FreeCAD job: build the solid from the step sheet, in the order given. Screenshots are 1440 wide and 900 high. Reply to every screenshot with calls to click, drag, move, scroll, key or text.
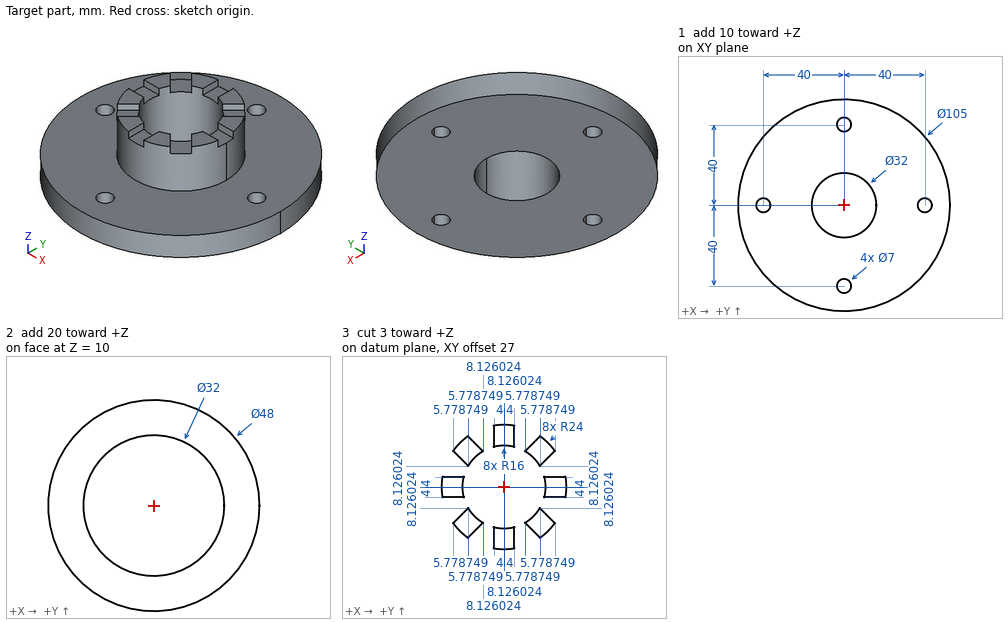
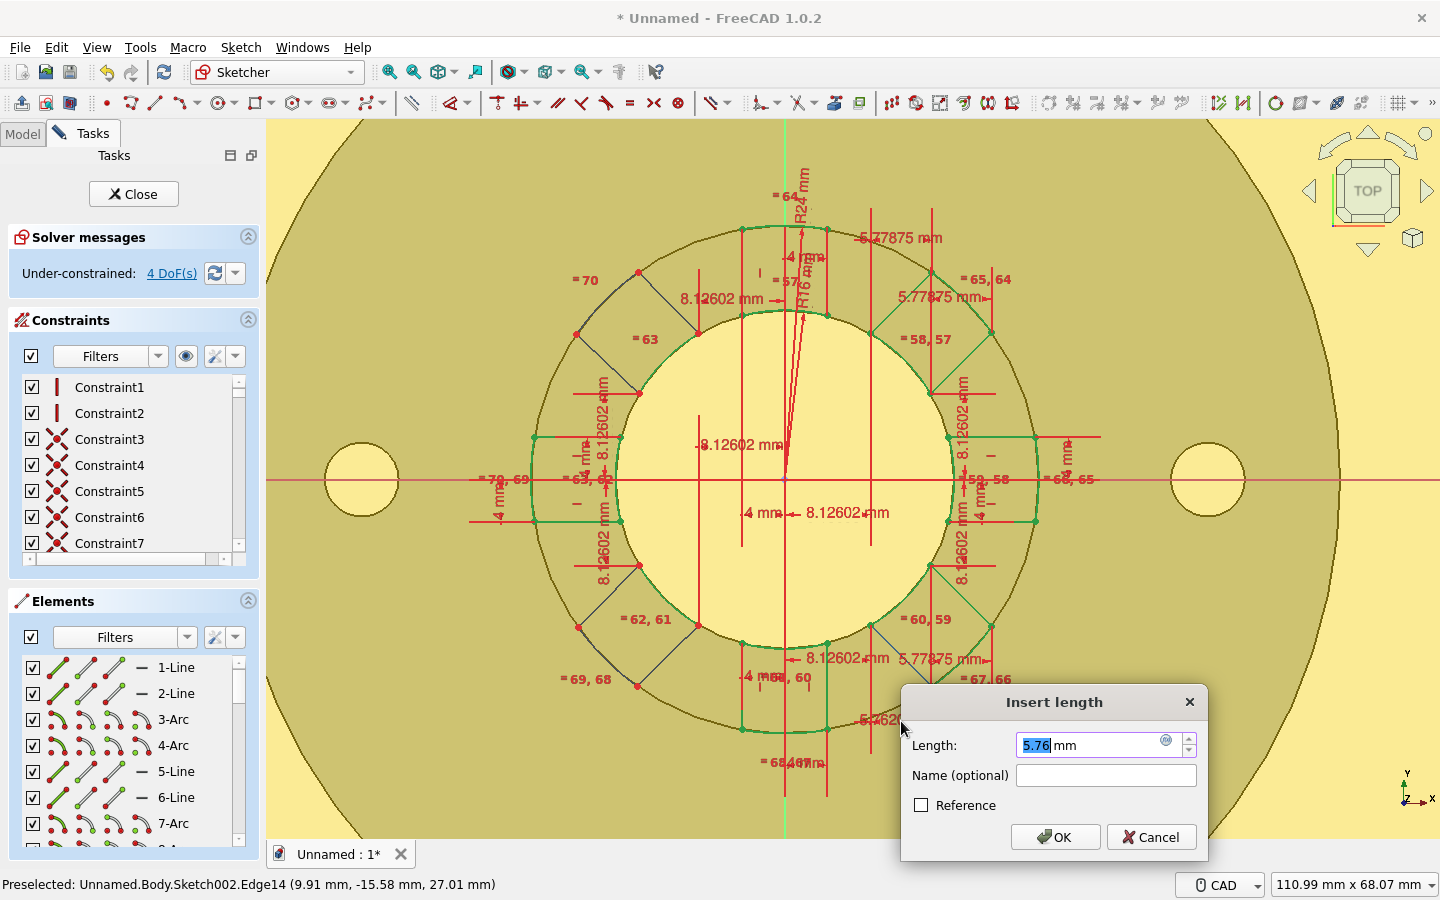
text(5.778749)
key(Return)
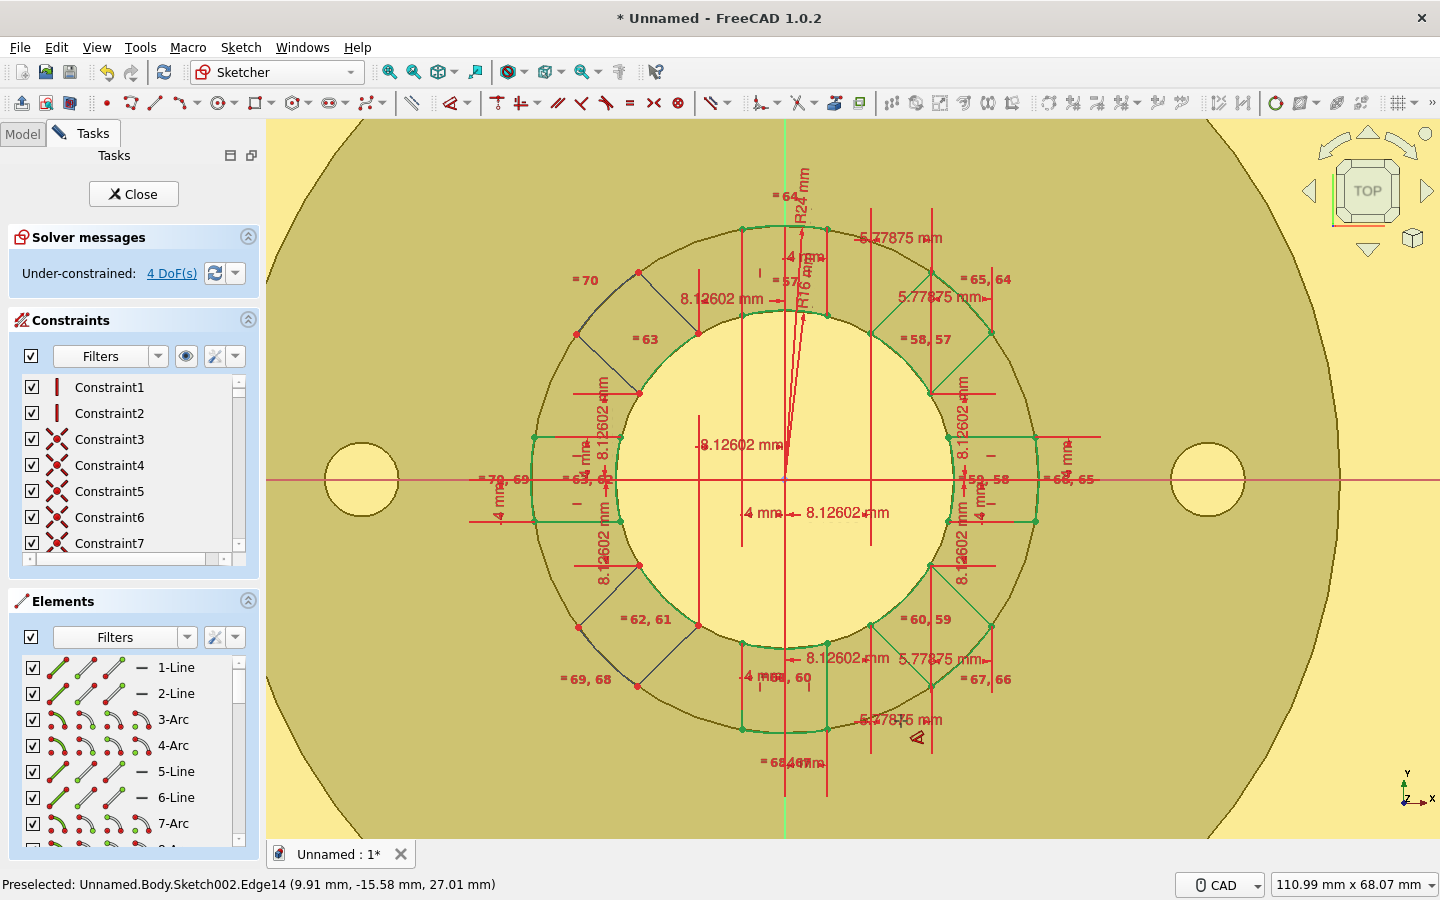
click(656, 668)
click(668, 720)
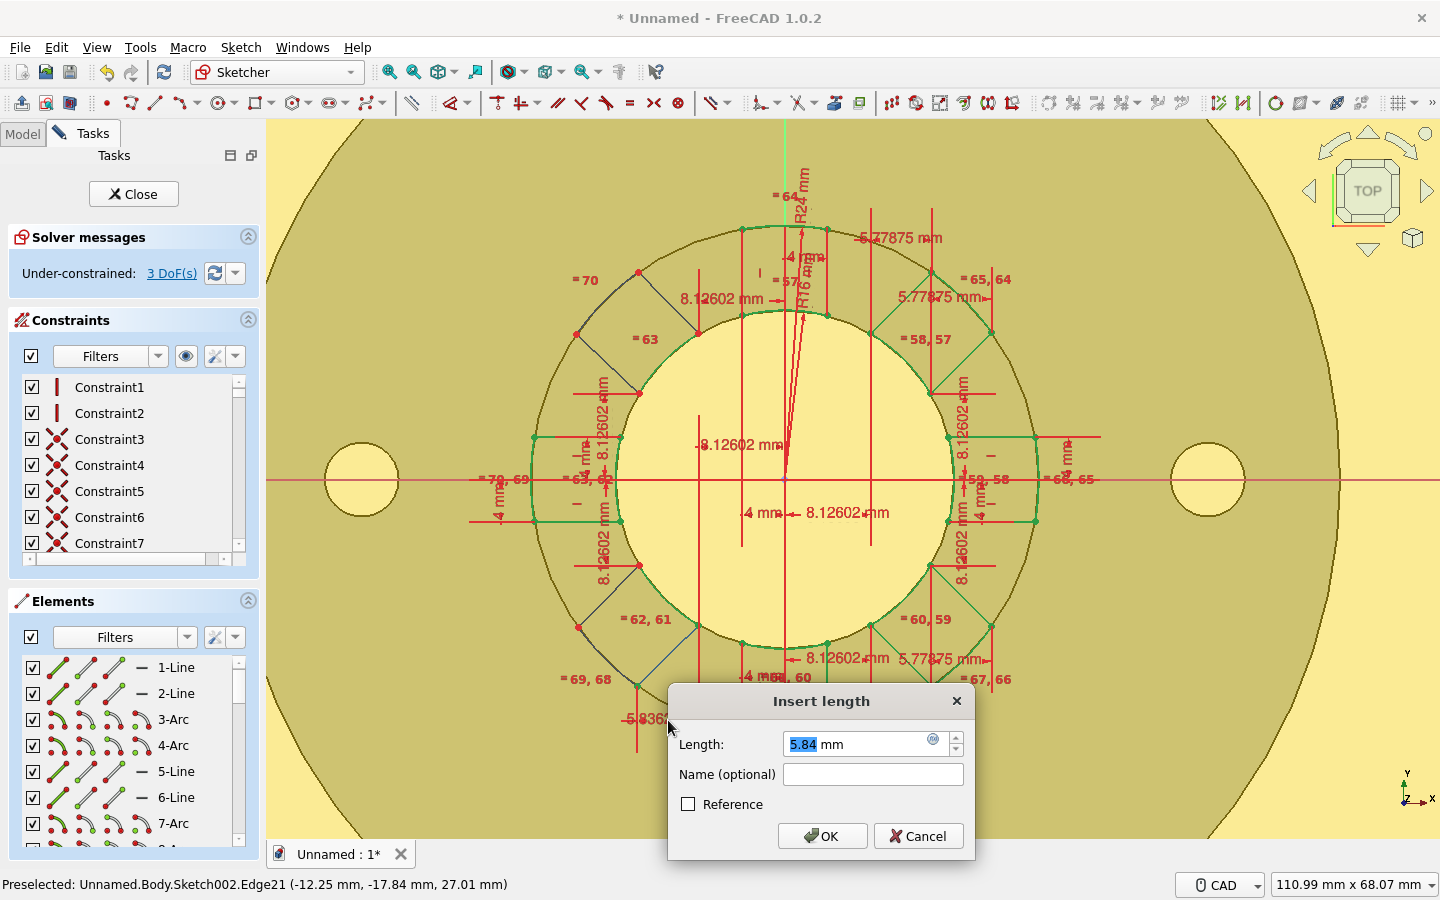
text(5.778749)
key(Return)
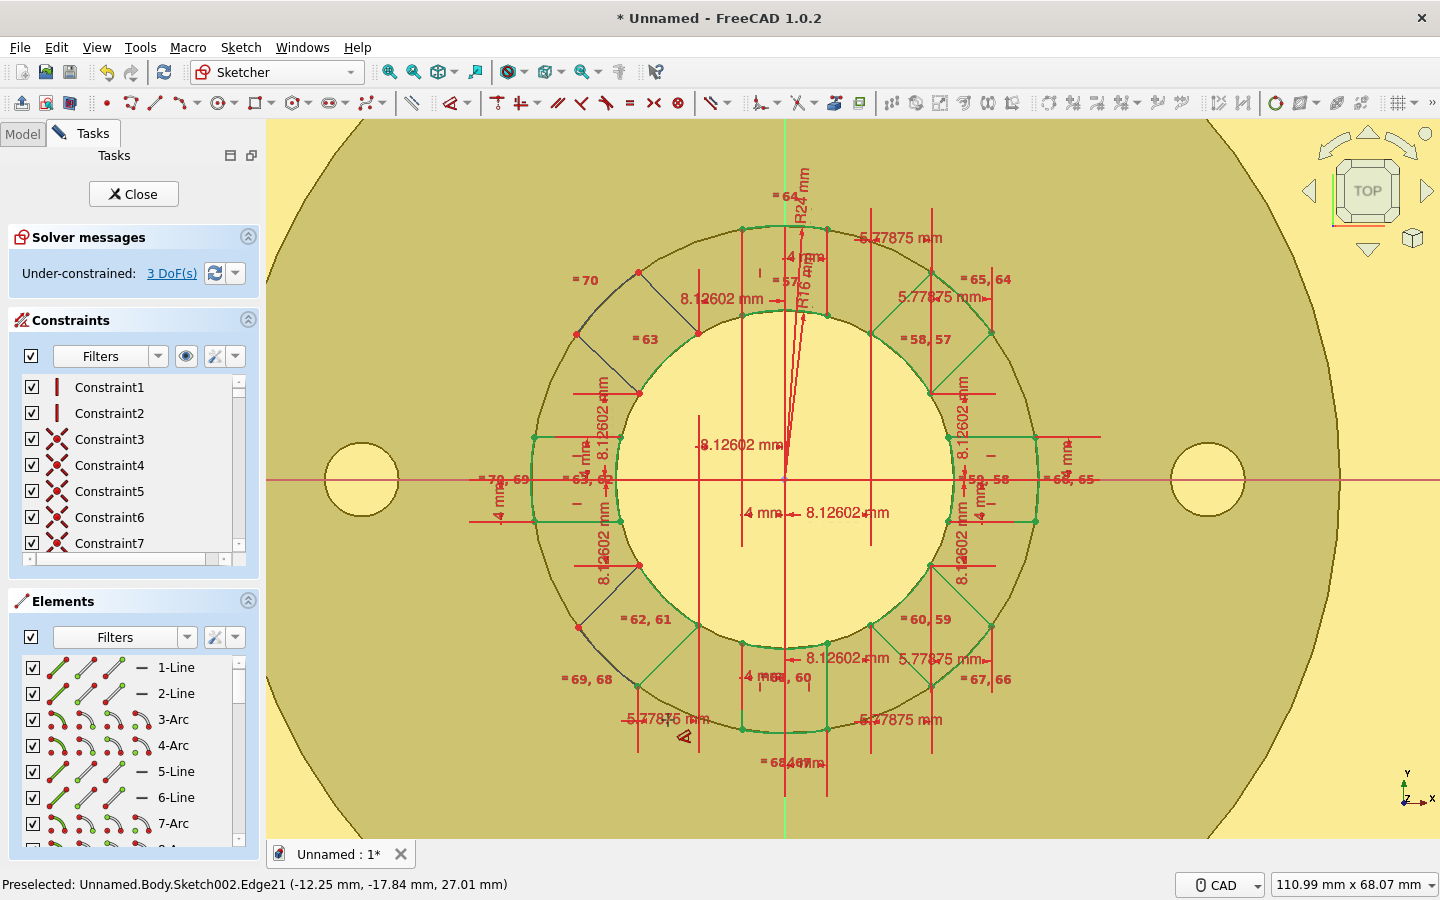
click(621, 584)
click(587, 661)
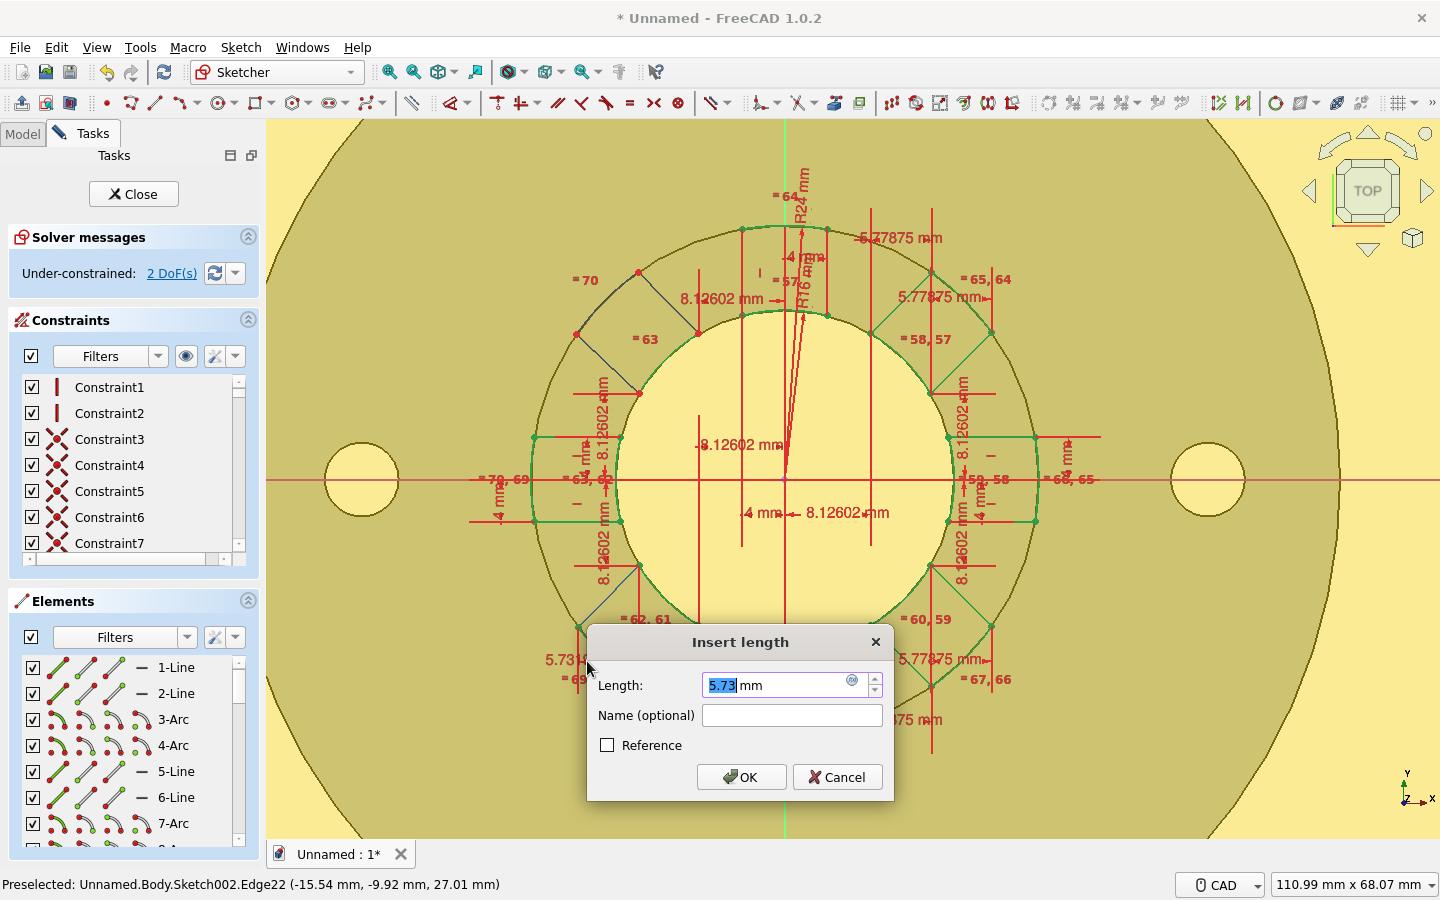
text(5.778749)
key(Return)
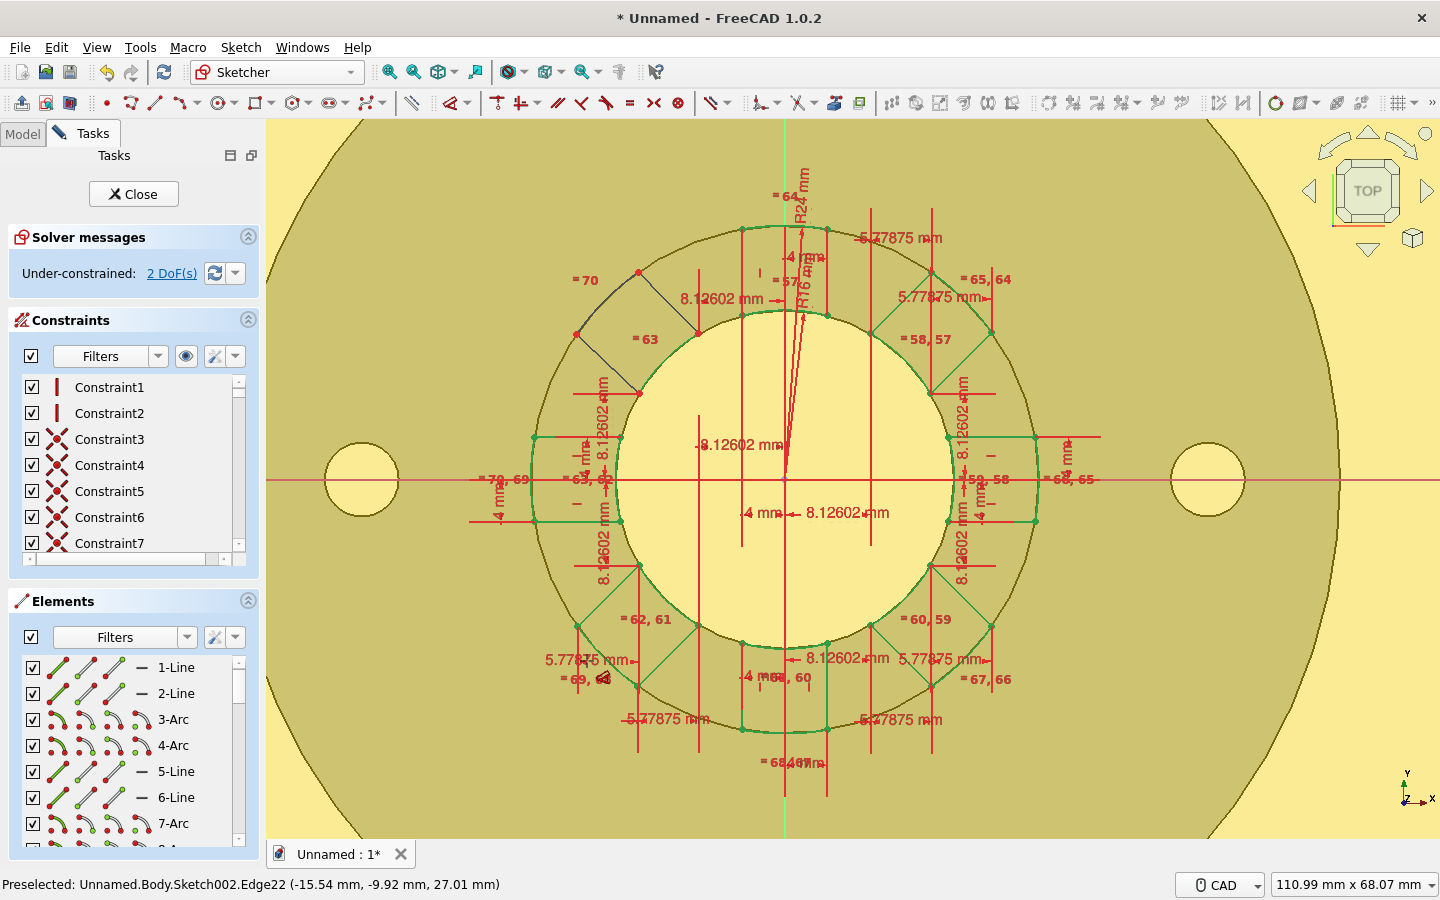
click(595, 352)
click(586, 300)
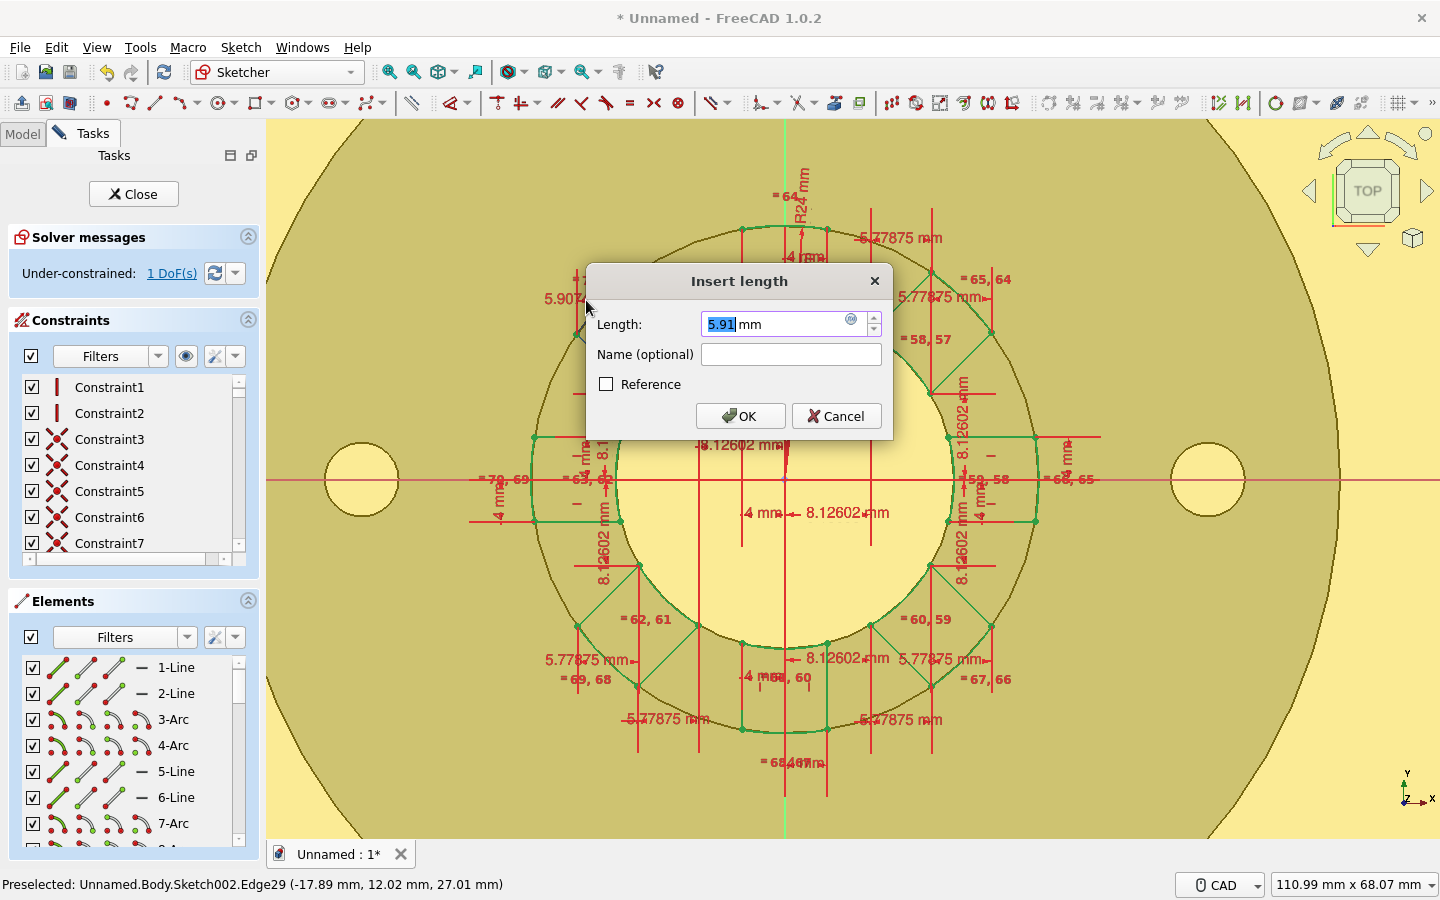
text(5.778749)
key(Return)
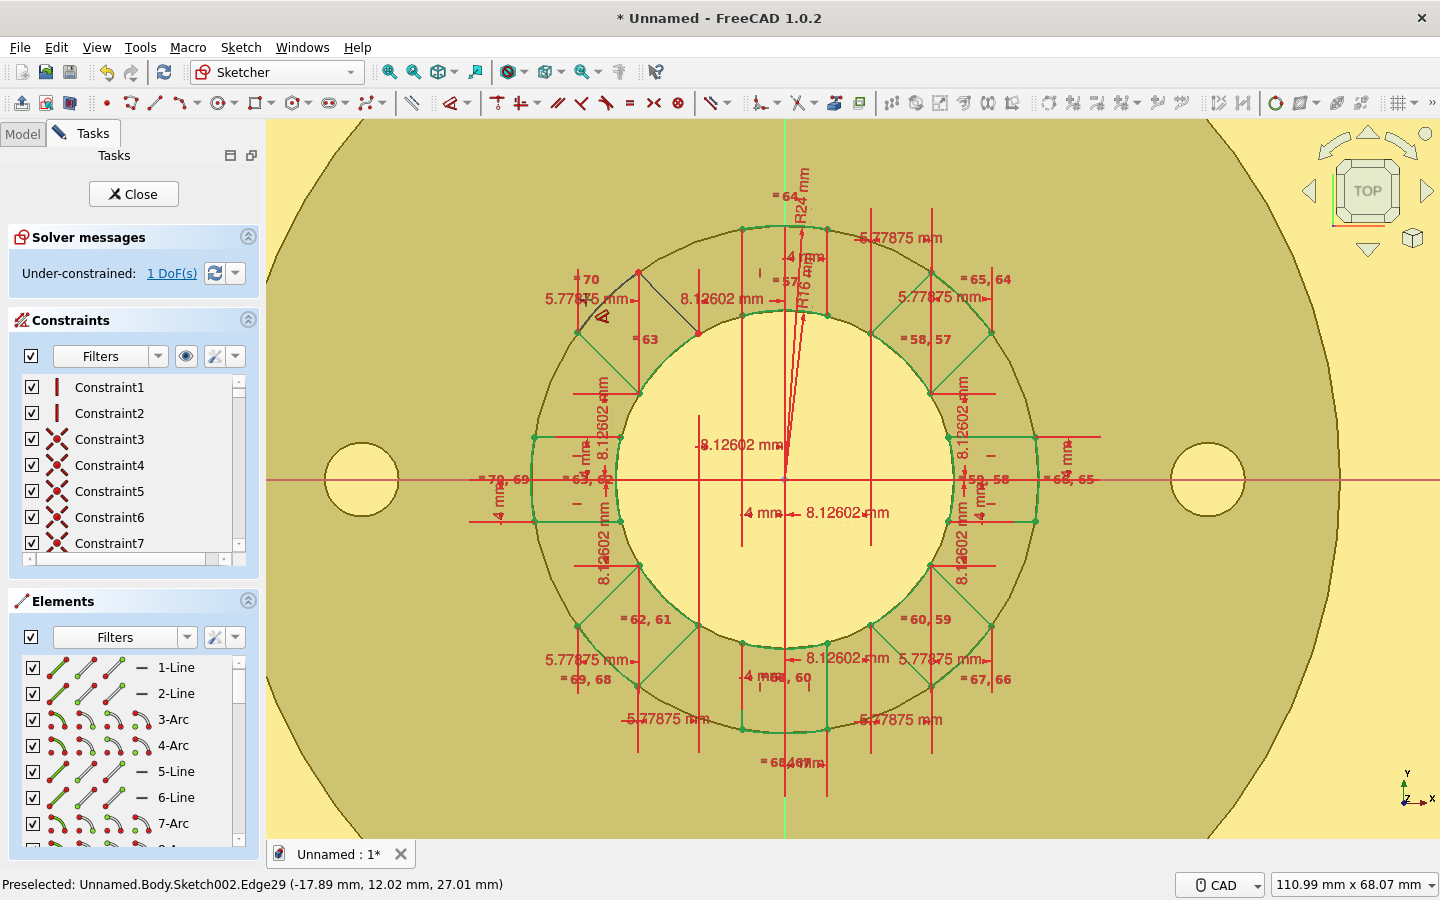
click(681, 315)
click(669, 238)